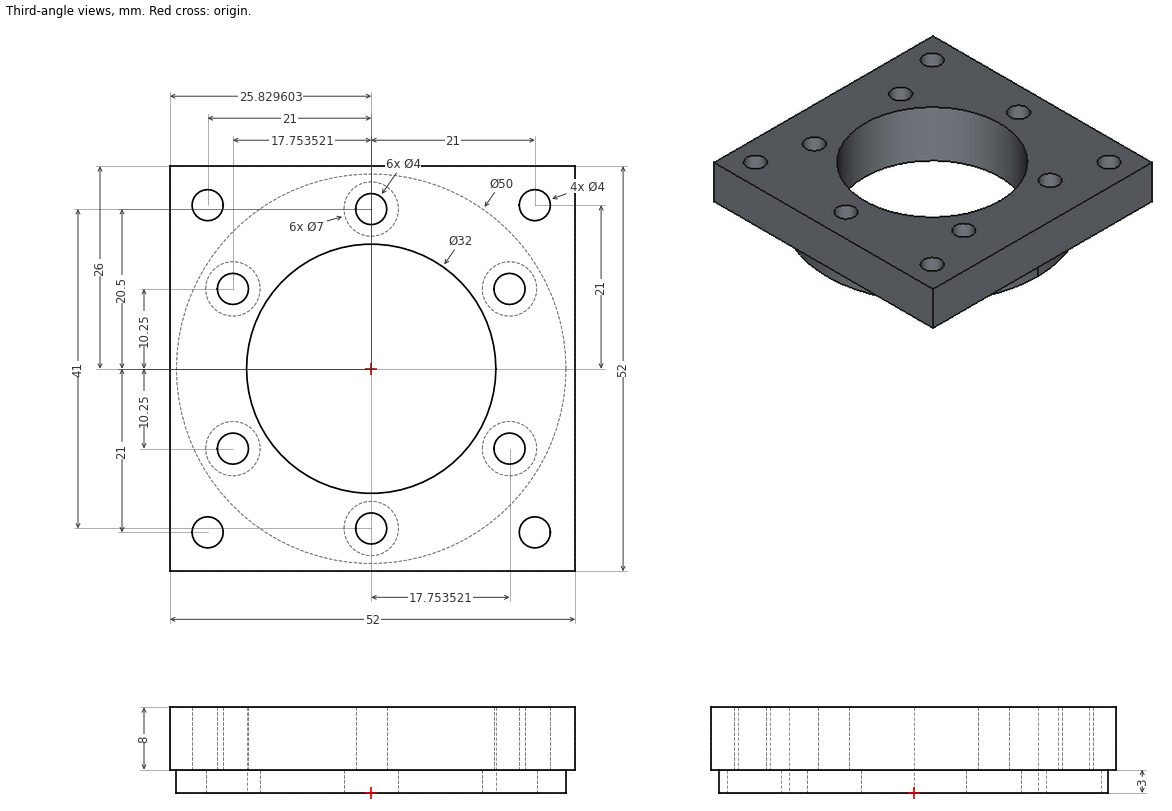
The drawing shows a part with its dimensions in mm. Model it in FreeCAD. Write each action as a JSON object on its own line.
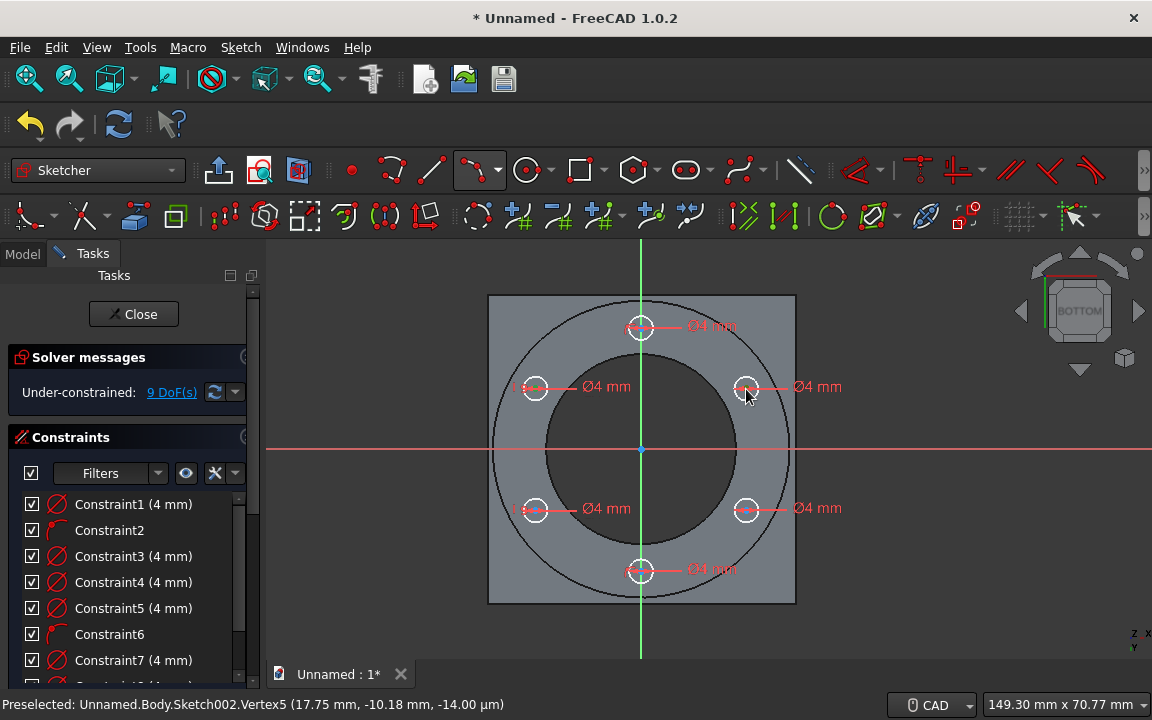
{"action": "key", "text": "h"}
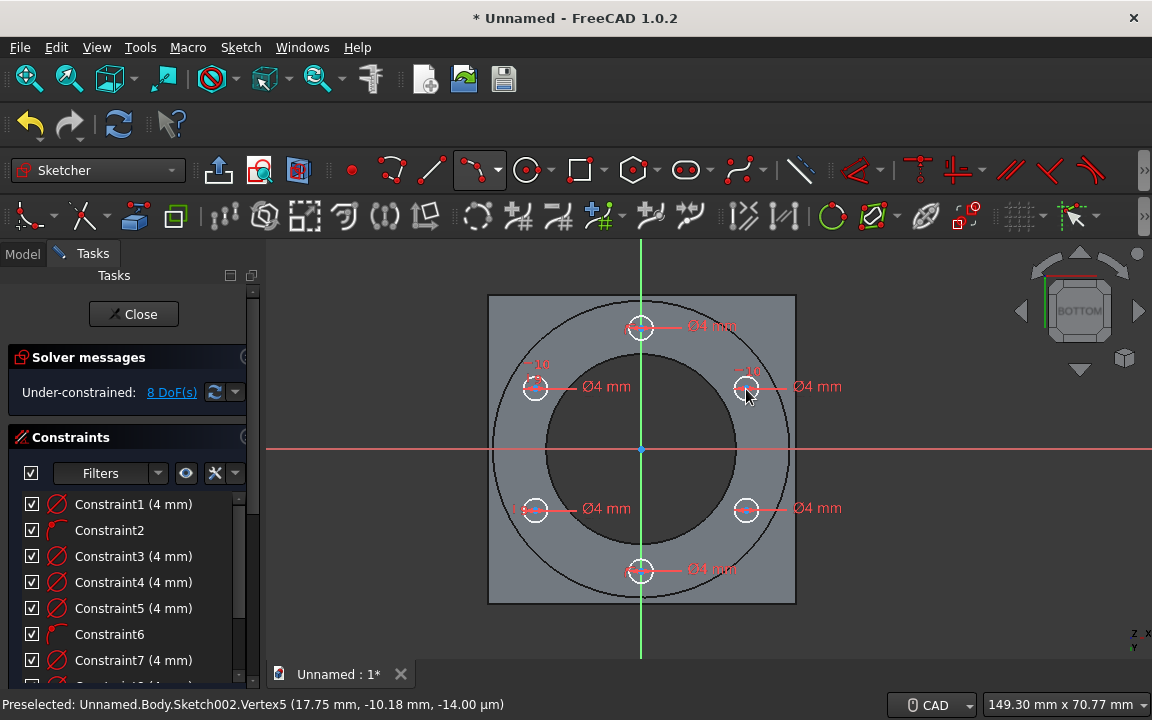
{"action": "left_click", "coordinate": [746, 389]}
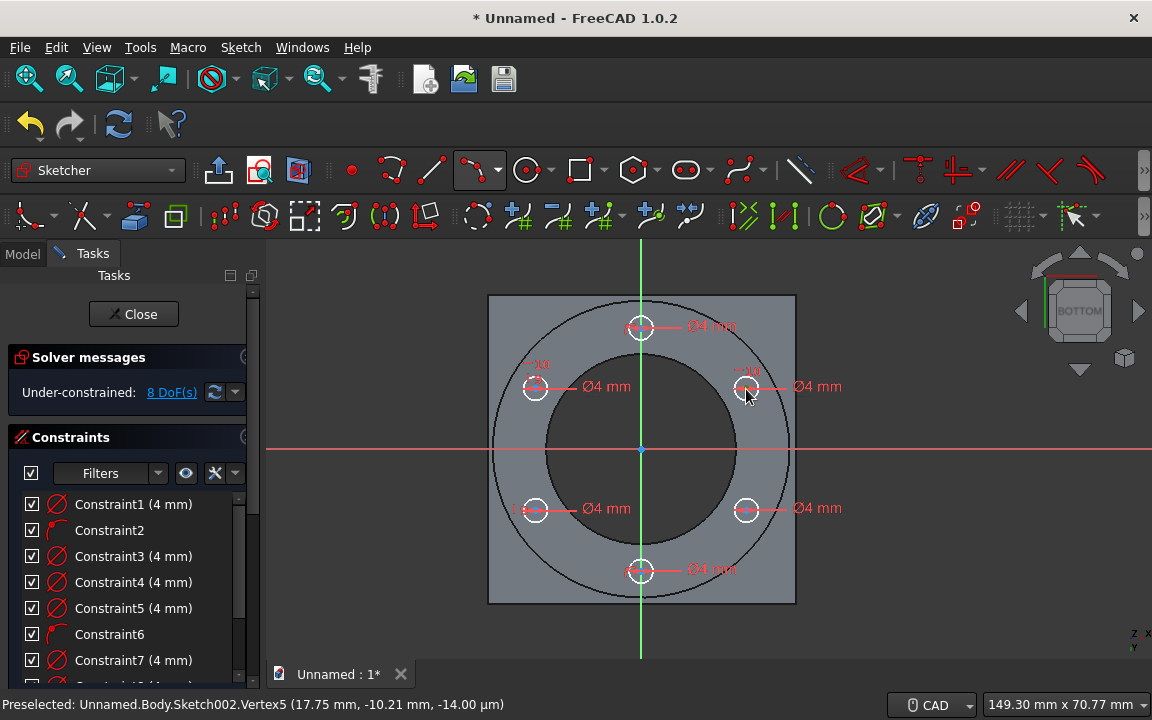
{"action": "left_click", "coordinate": [746, 510]}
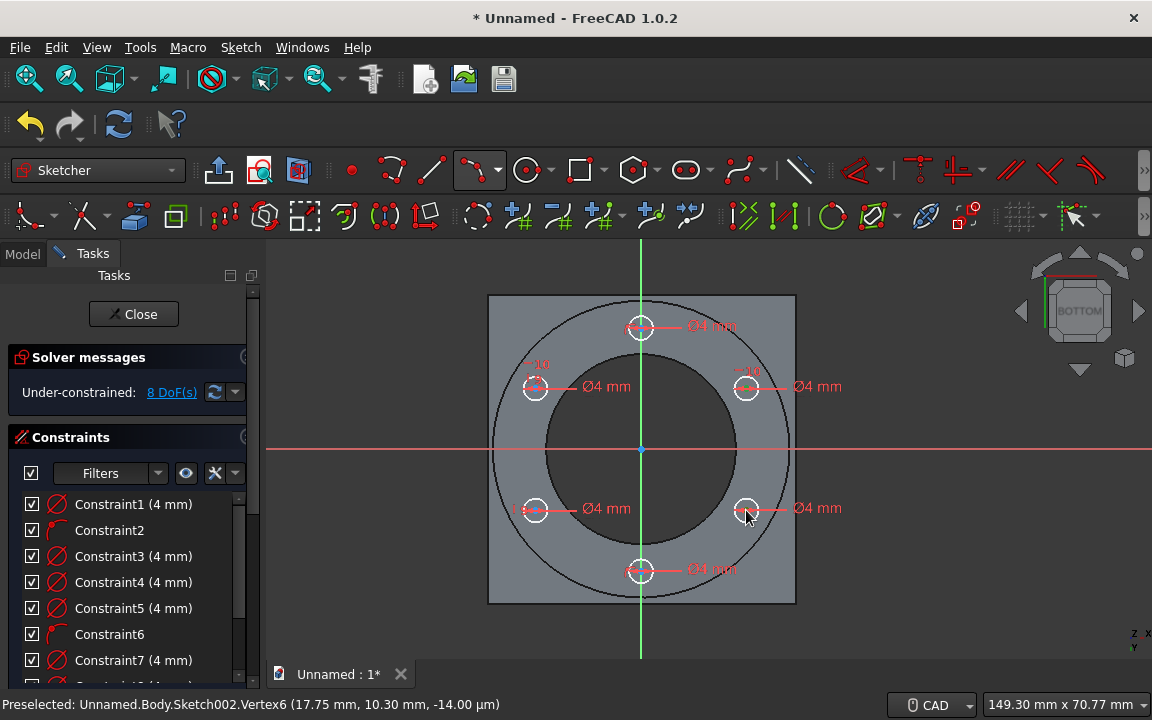
{"action": "left_click", "coordinate": [984, 170]}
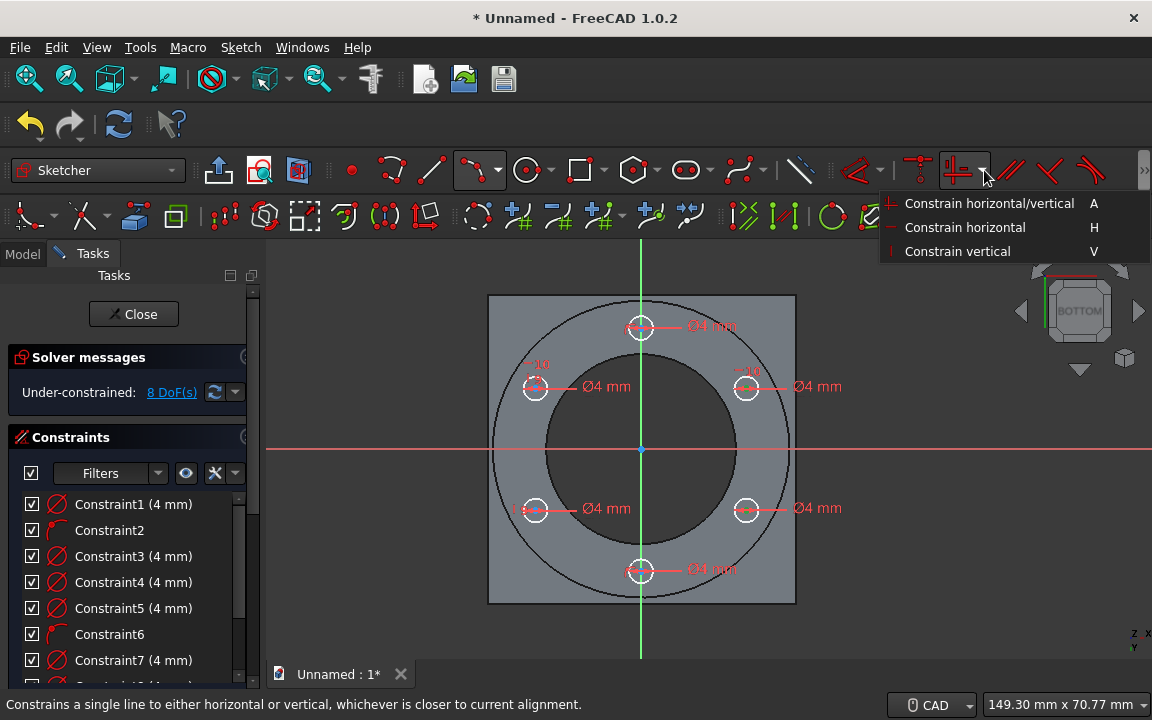
{"action": "left_click", "coordinate": [1015, 251]}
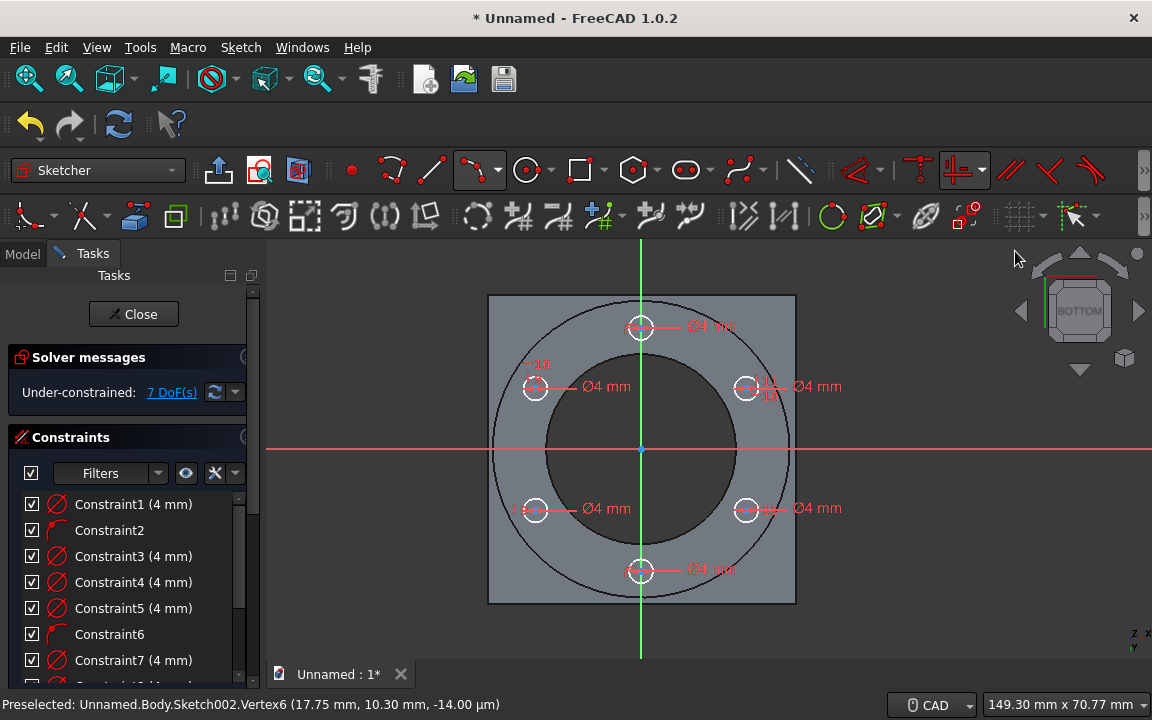
{"action": "left_click", "coordinate": [536, 511]}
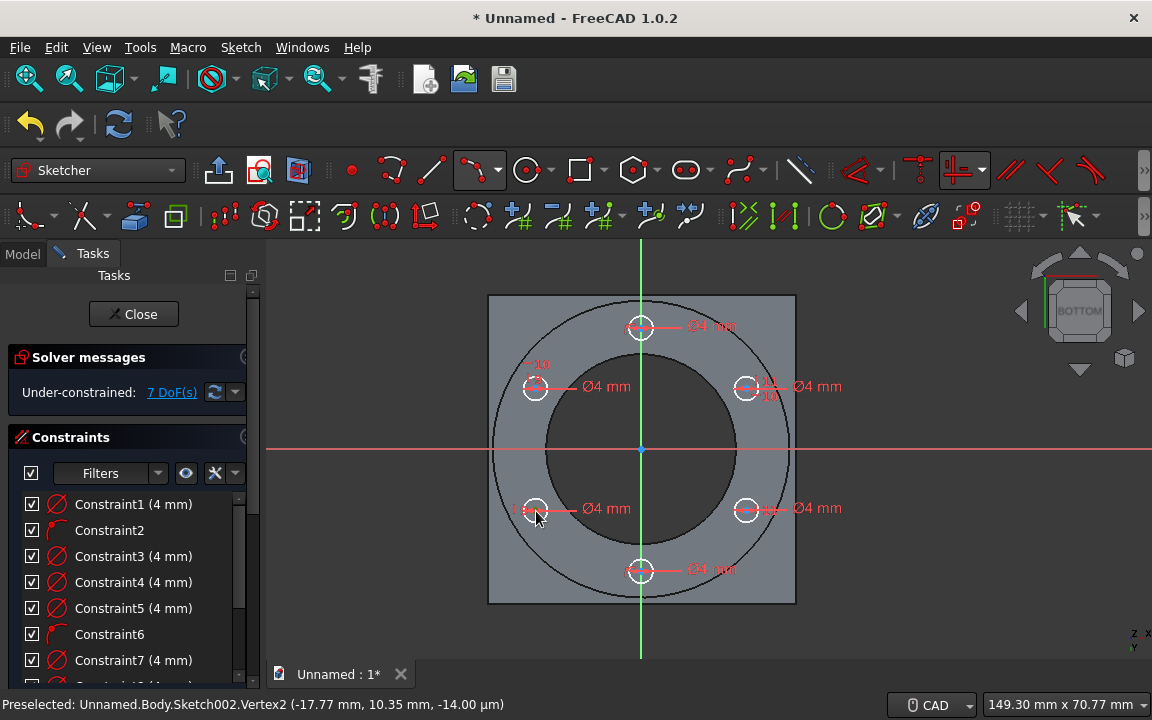
{"action": "left_click", "coordinate": [746, 510]}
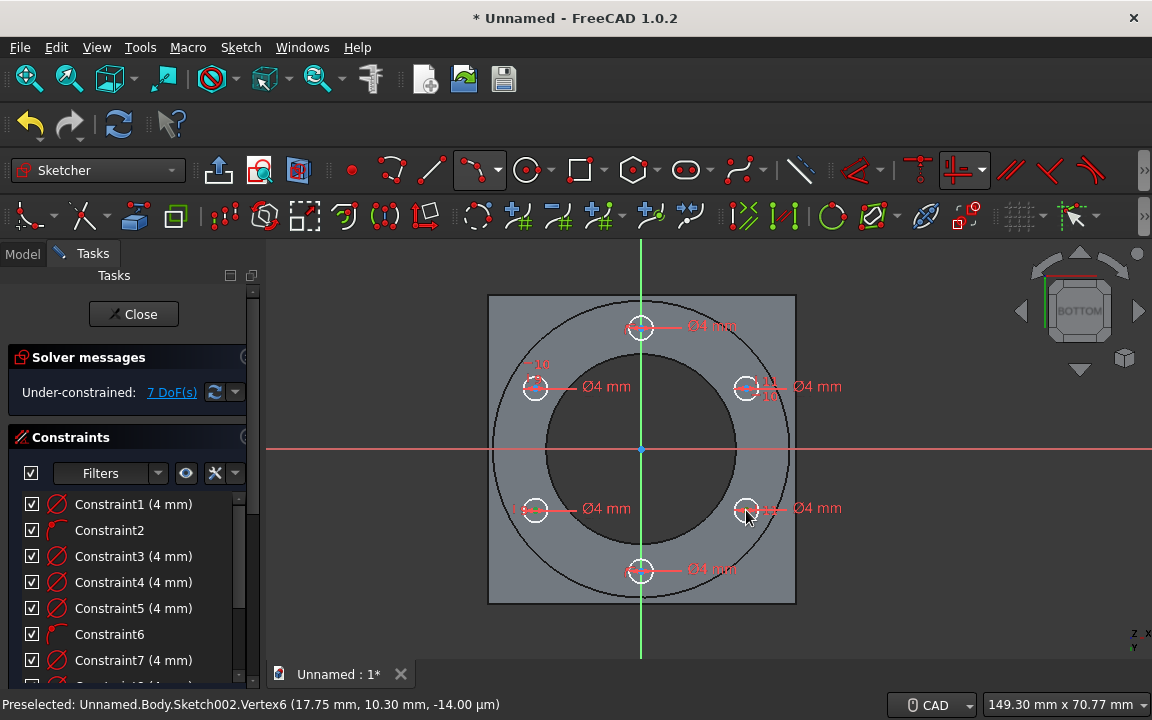
{"action": "key", "text": "h"}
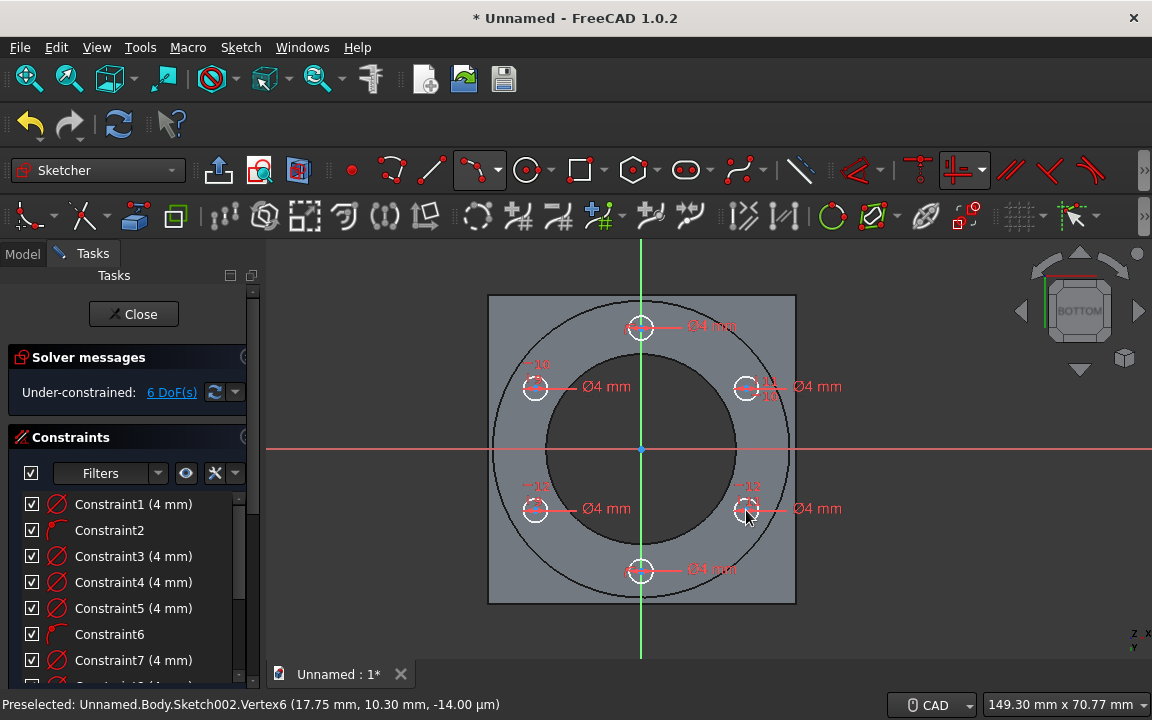
{"action": "left_click", "coordinate": [856, 170]}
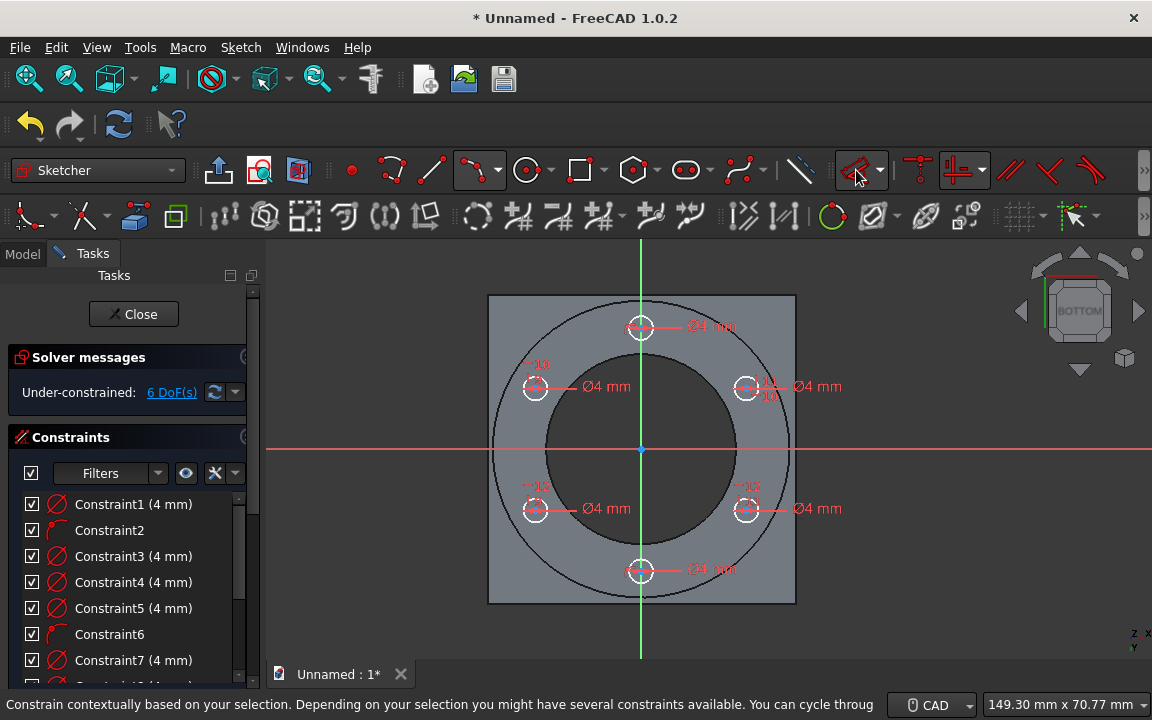
{"action": "left_click", "coordinate": [641, 571]}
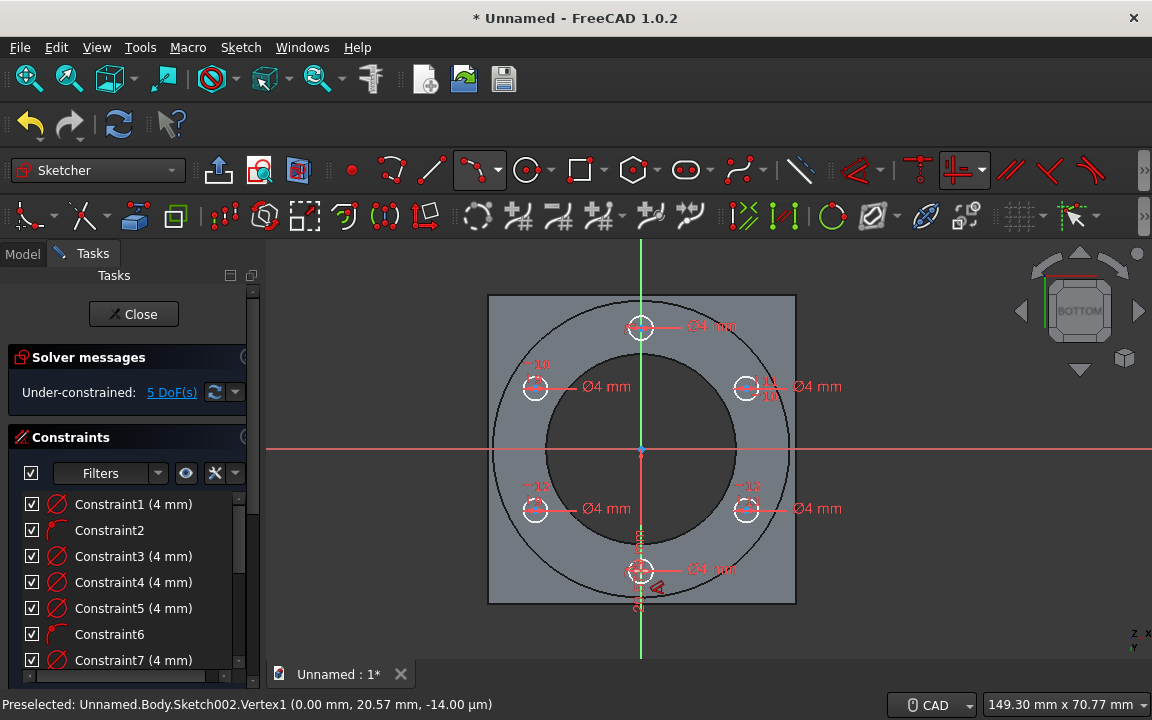
{"action": "left_click", "coordinate": [641, 328]}
{"action": "left_click", "coordinate": [675, 394]}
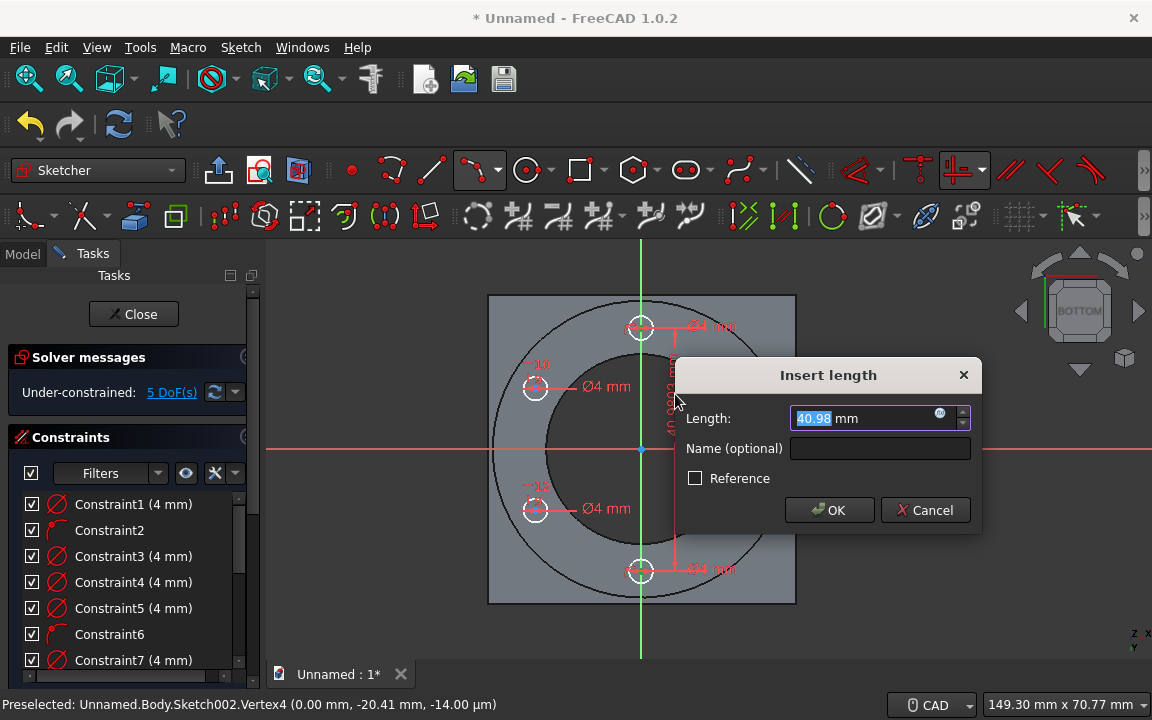
{"action": "type", "text": "41"}
{"action": "key", "text": "Return"}